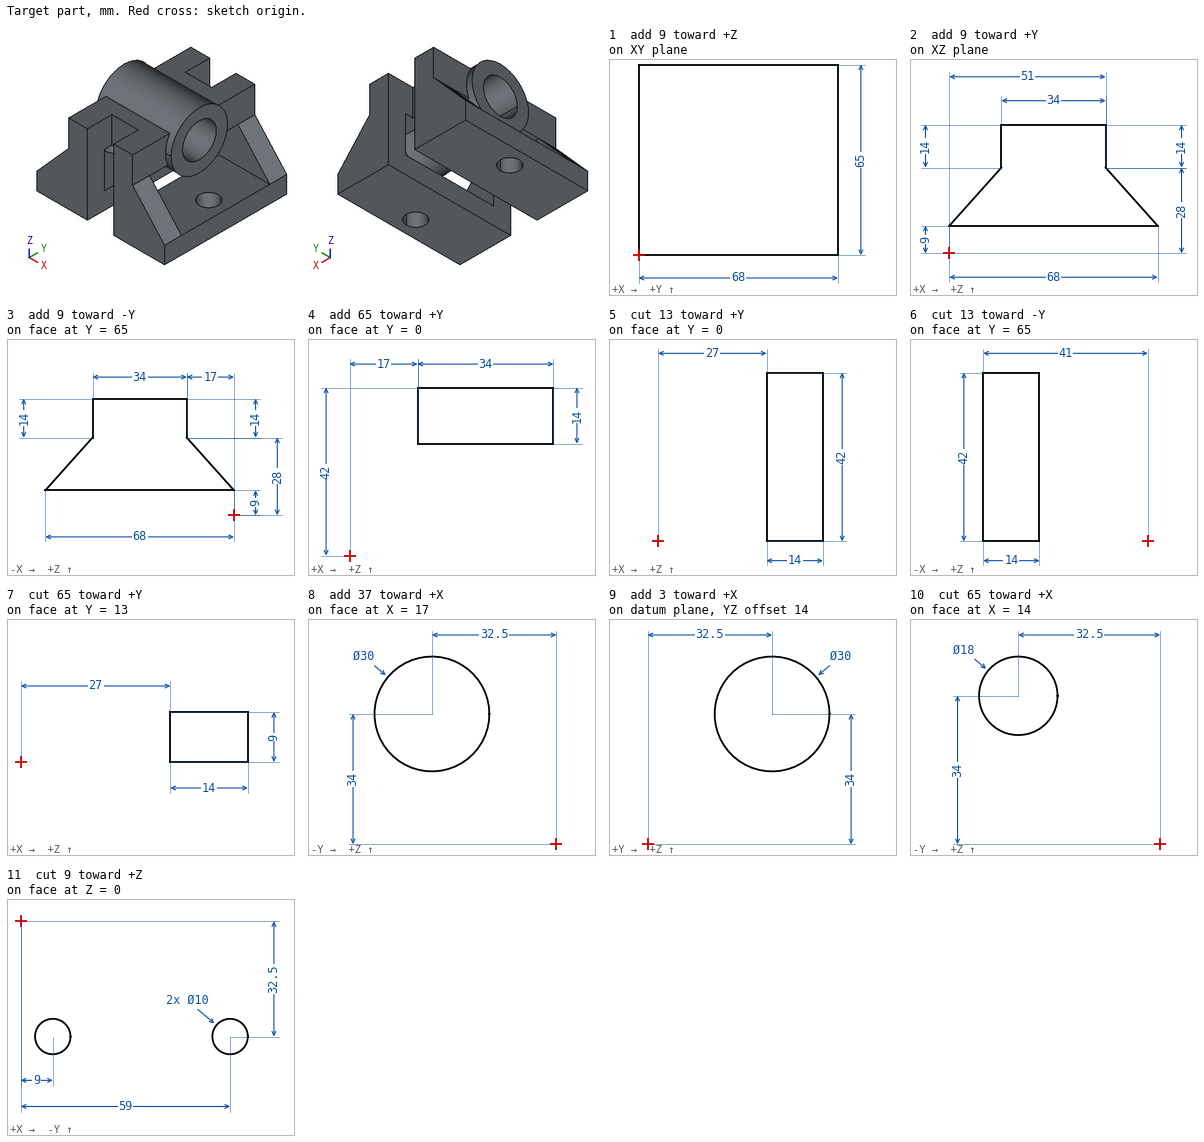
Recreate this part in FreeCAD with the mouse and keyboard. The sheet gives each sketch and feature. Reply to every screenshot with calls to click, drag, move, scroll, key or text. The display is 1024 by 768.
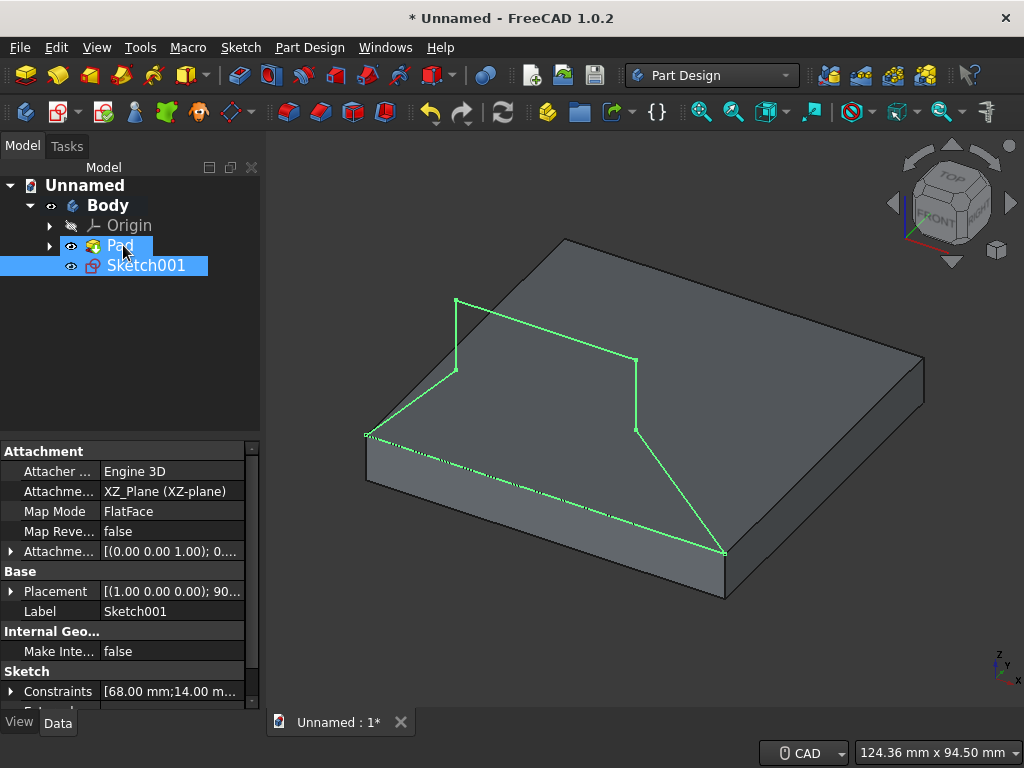
click(26, 76)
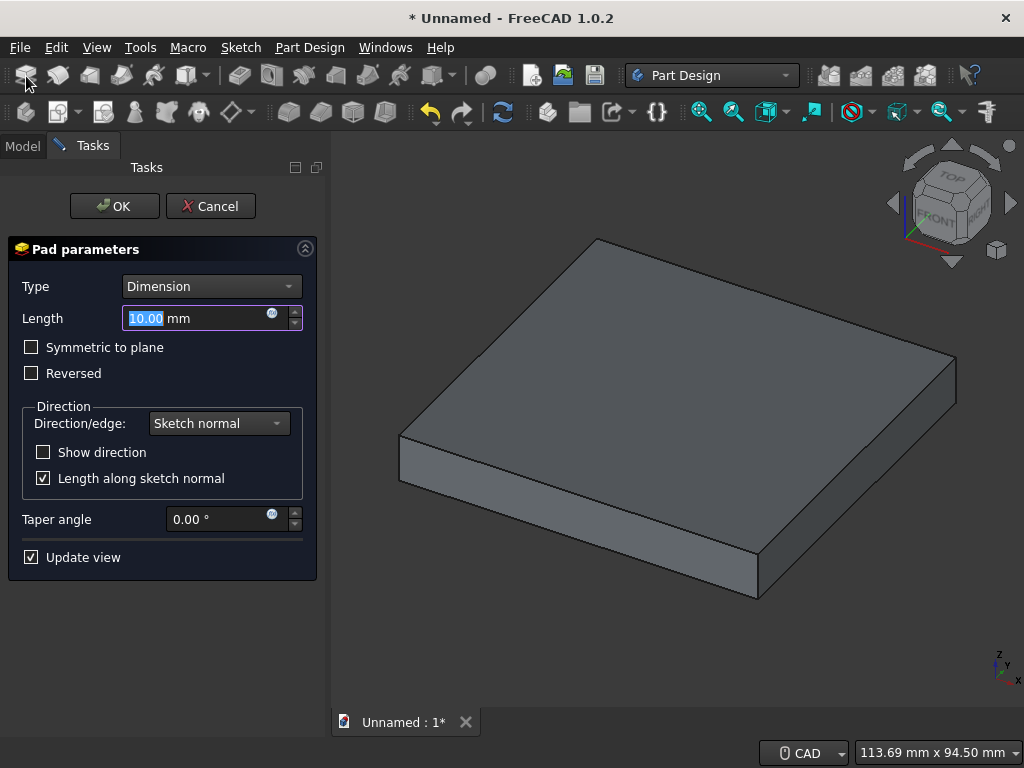
text(9)
key(Tab)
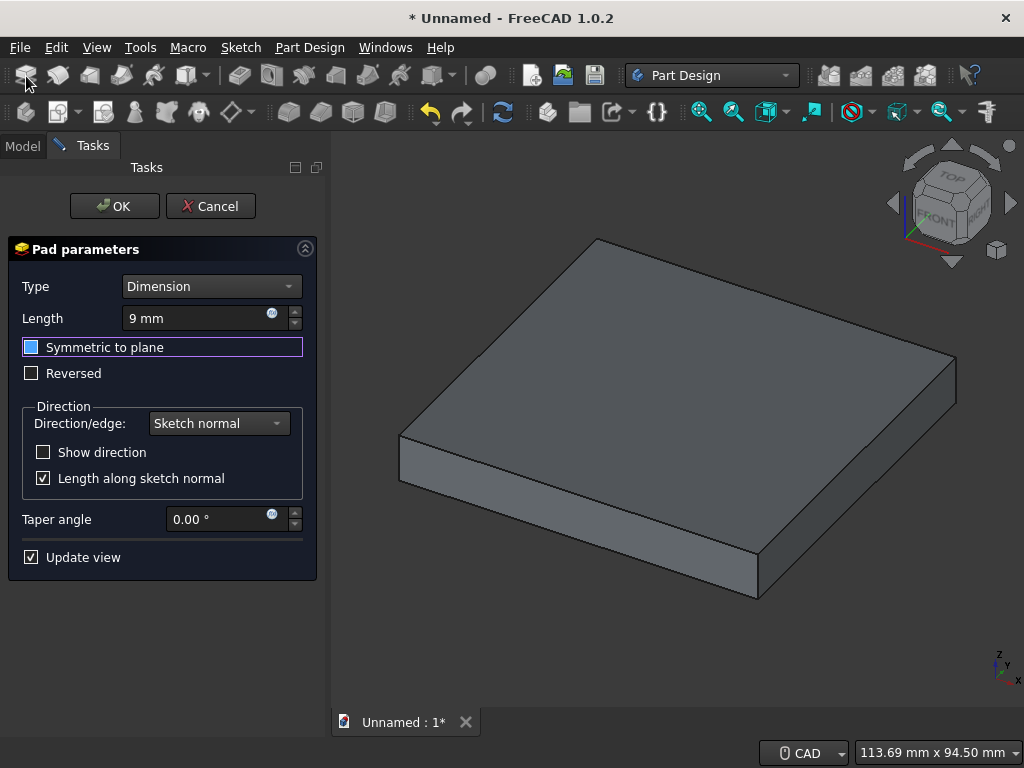
click(30, 373)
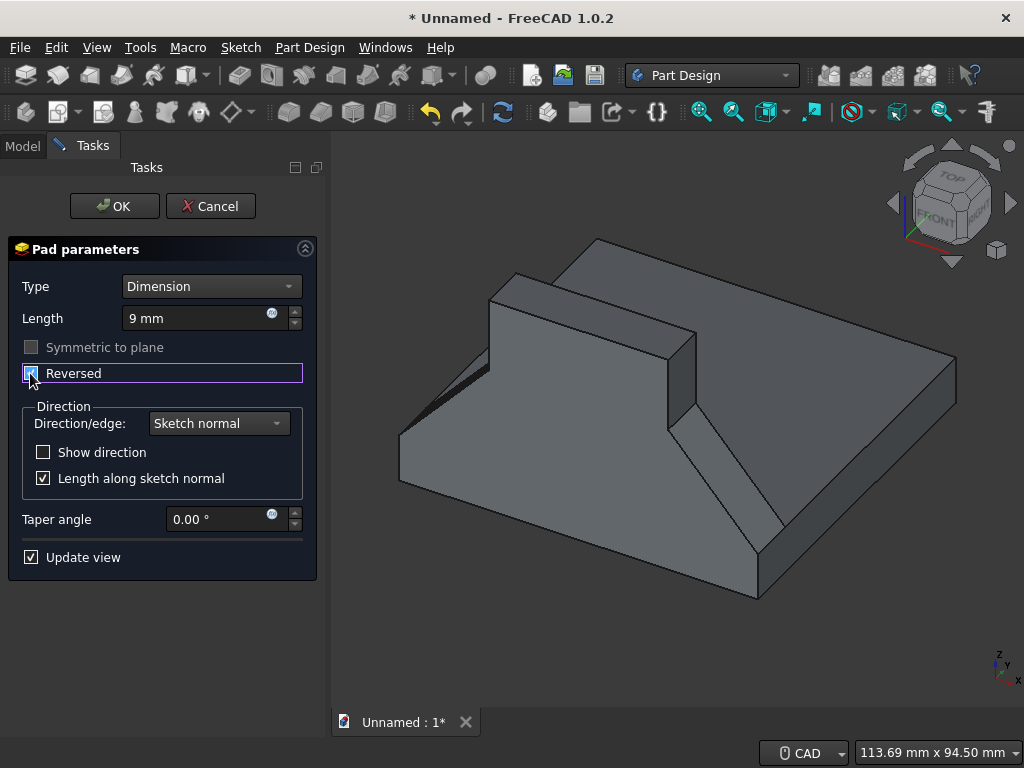
click(115, 206)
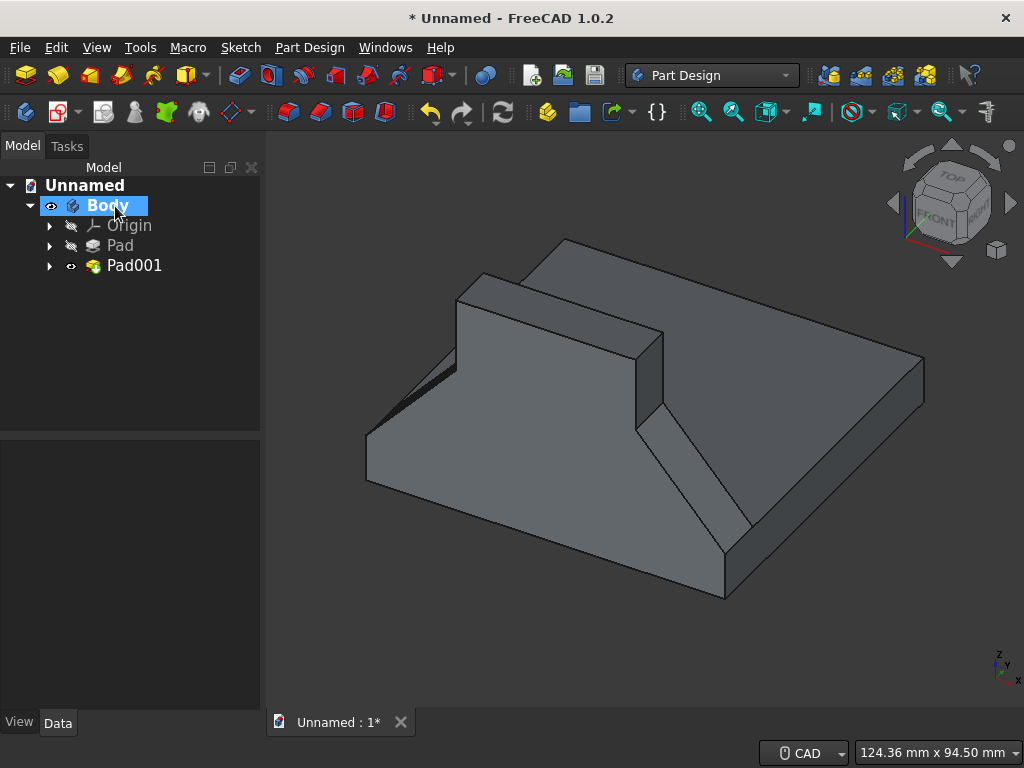
key(v)
key(f)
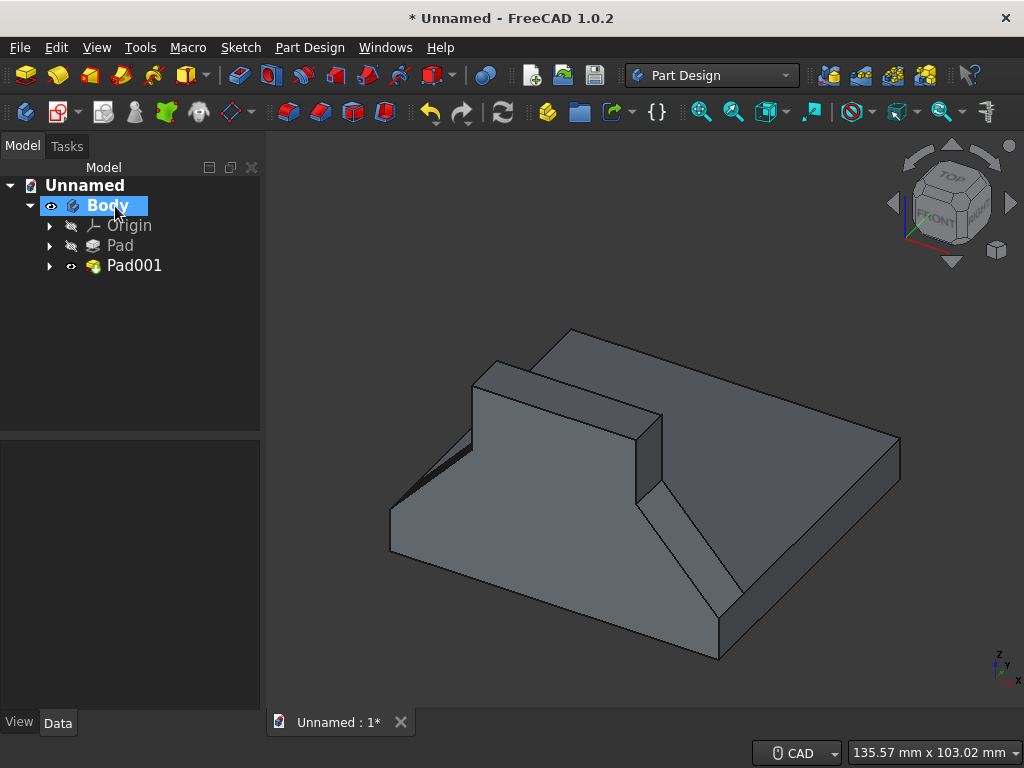
key(4)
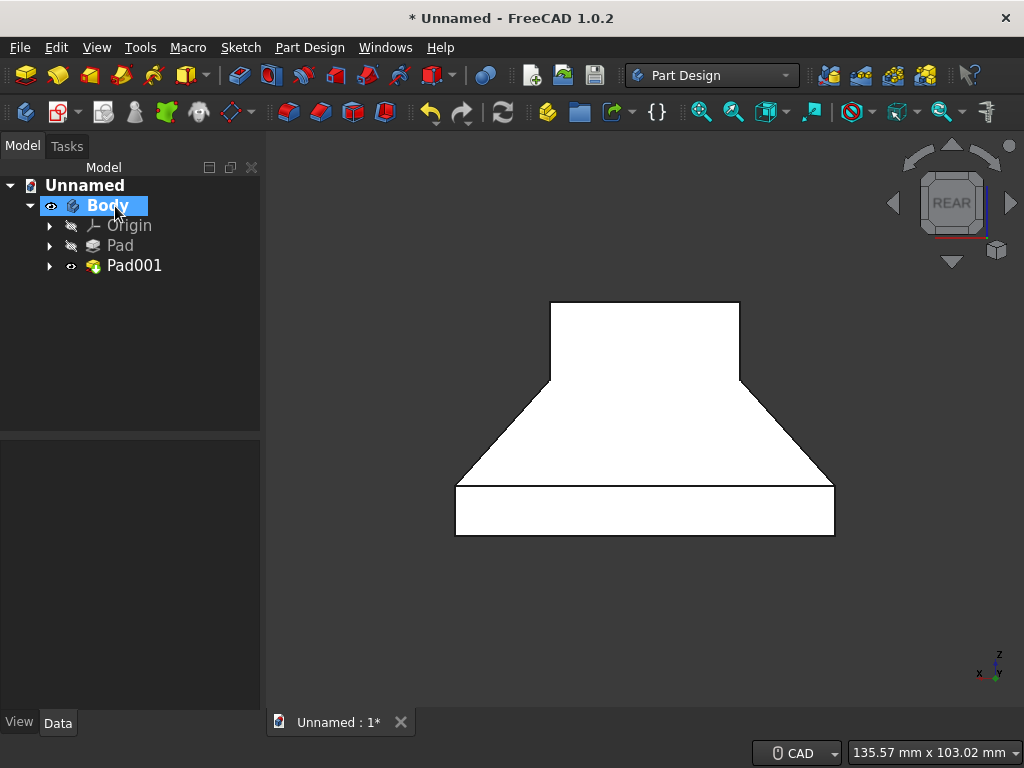
click(482, 510)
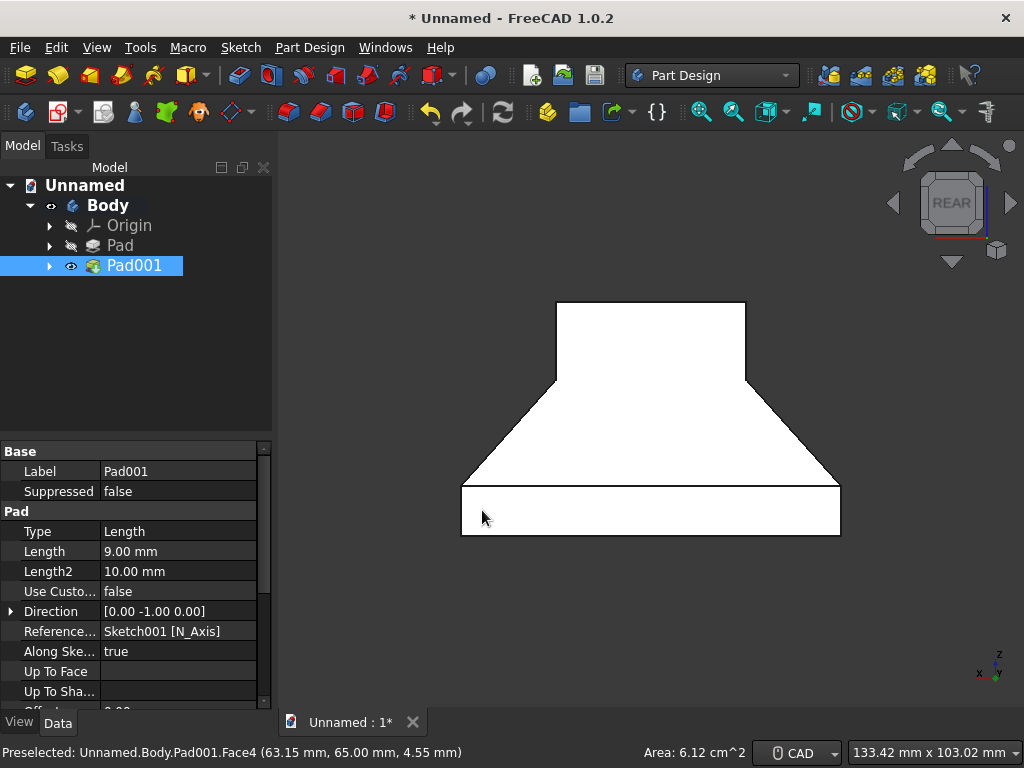
click(58, 112)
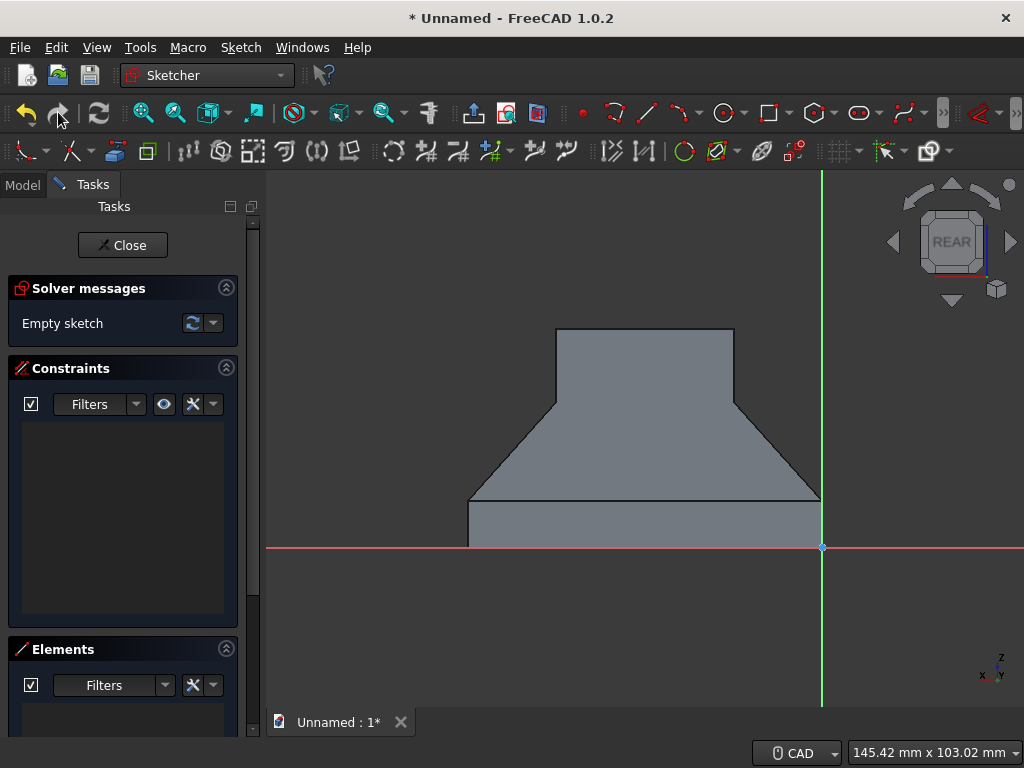
key(g)
key(m)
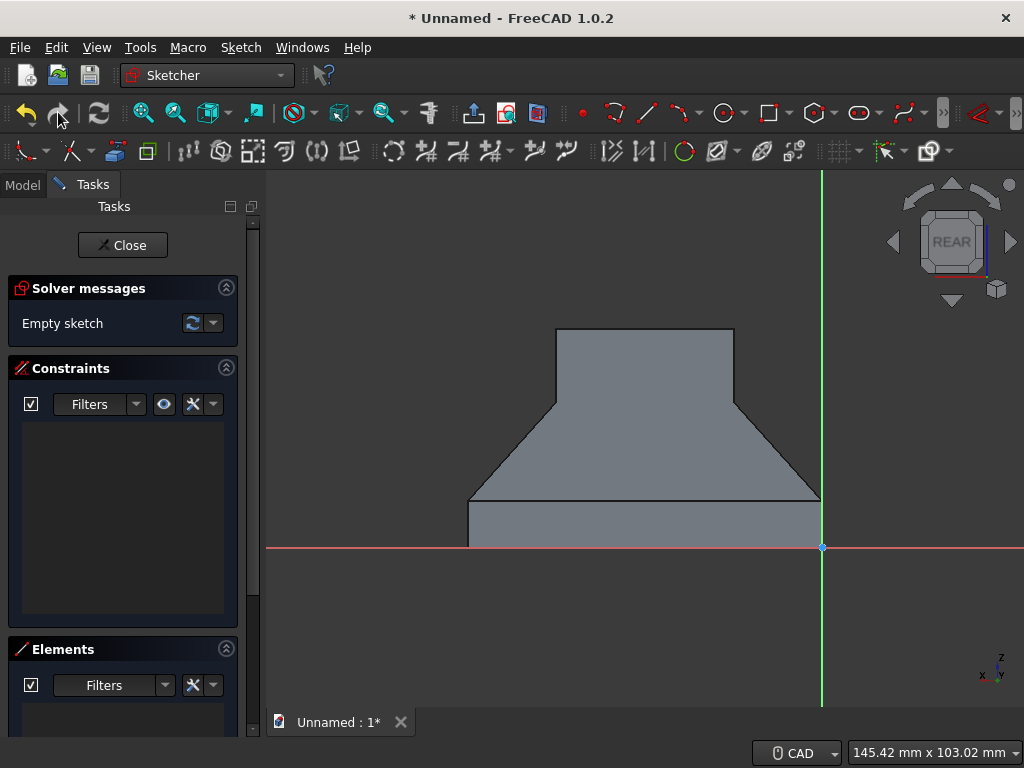
click(822, 501)
click(734, 402)
click(734, 329)
click(556, 329)
click(556, 402)
click(468, 501)
click(822, 502)
key(Escape)
key(Escape)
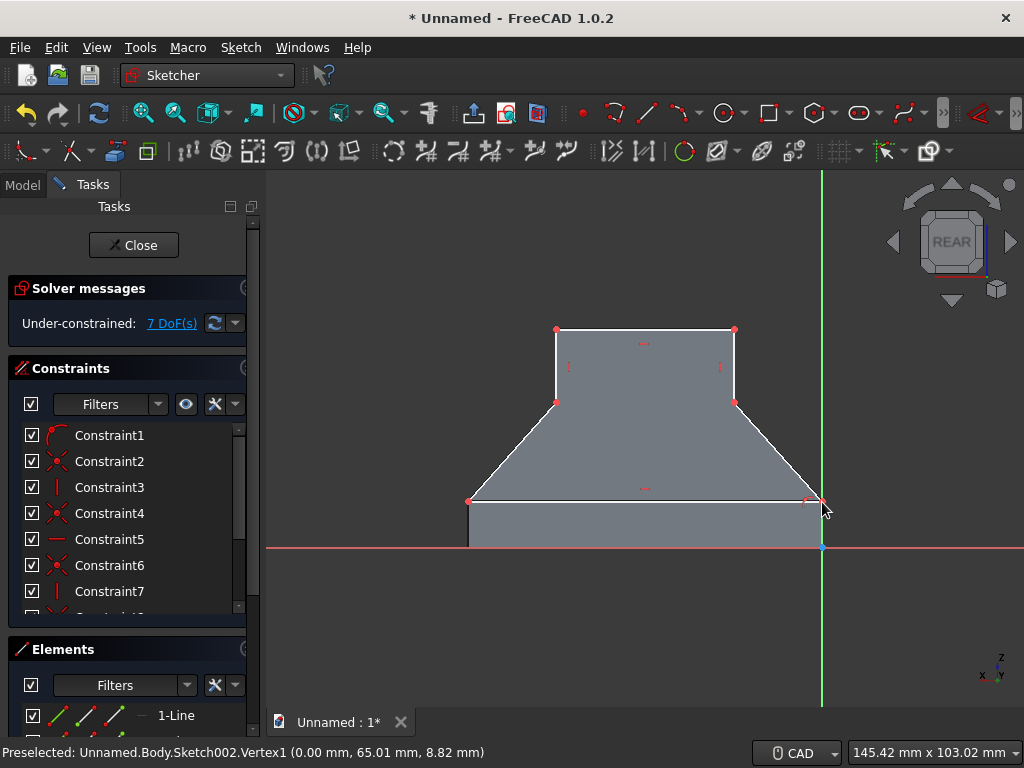
click(978, 114)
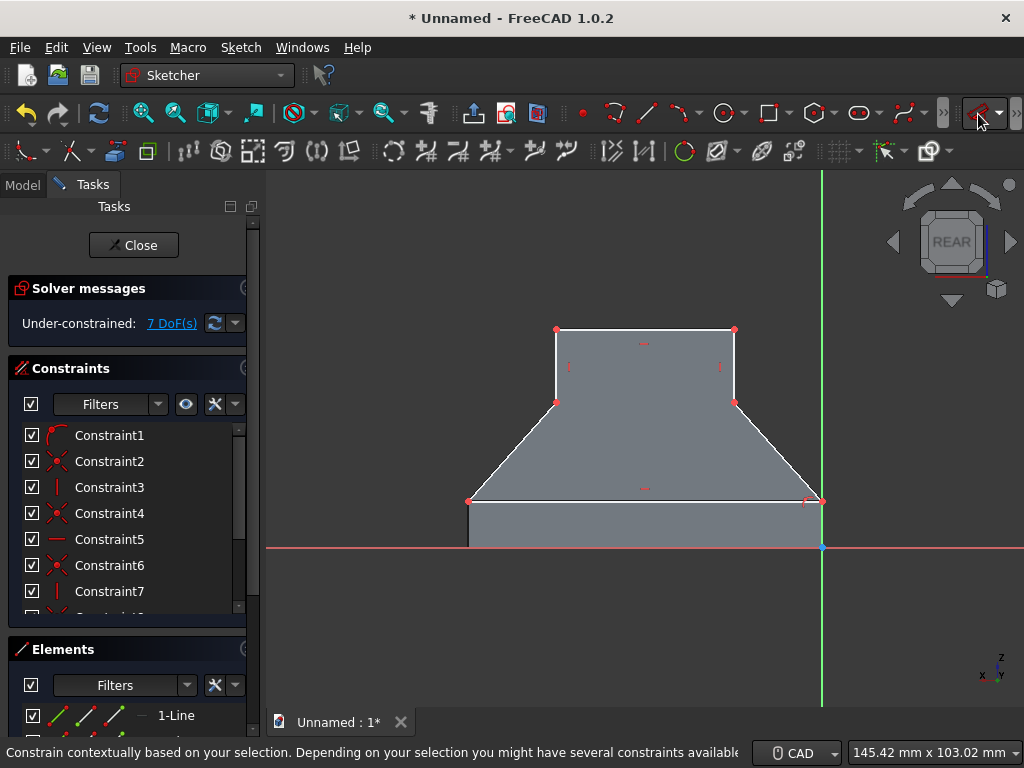
click(734, 381)
click(768, 367)